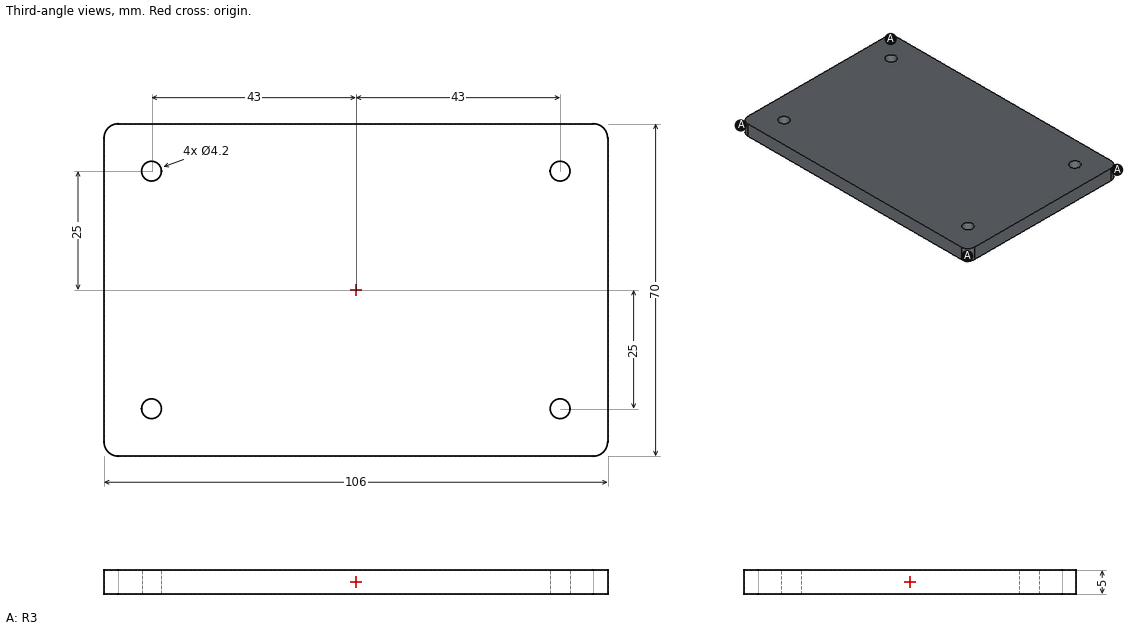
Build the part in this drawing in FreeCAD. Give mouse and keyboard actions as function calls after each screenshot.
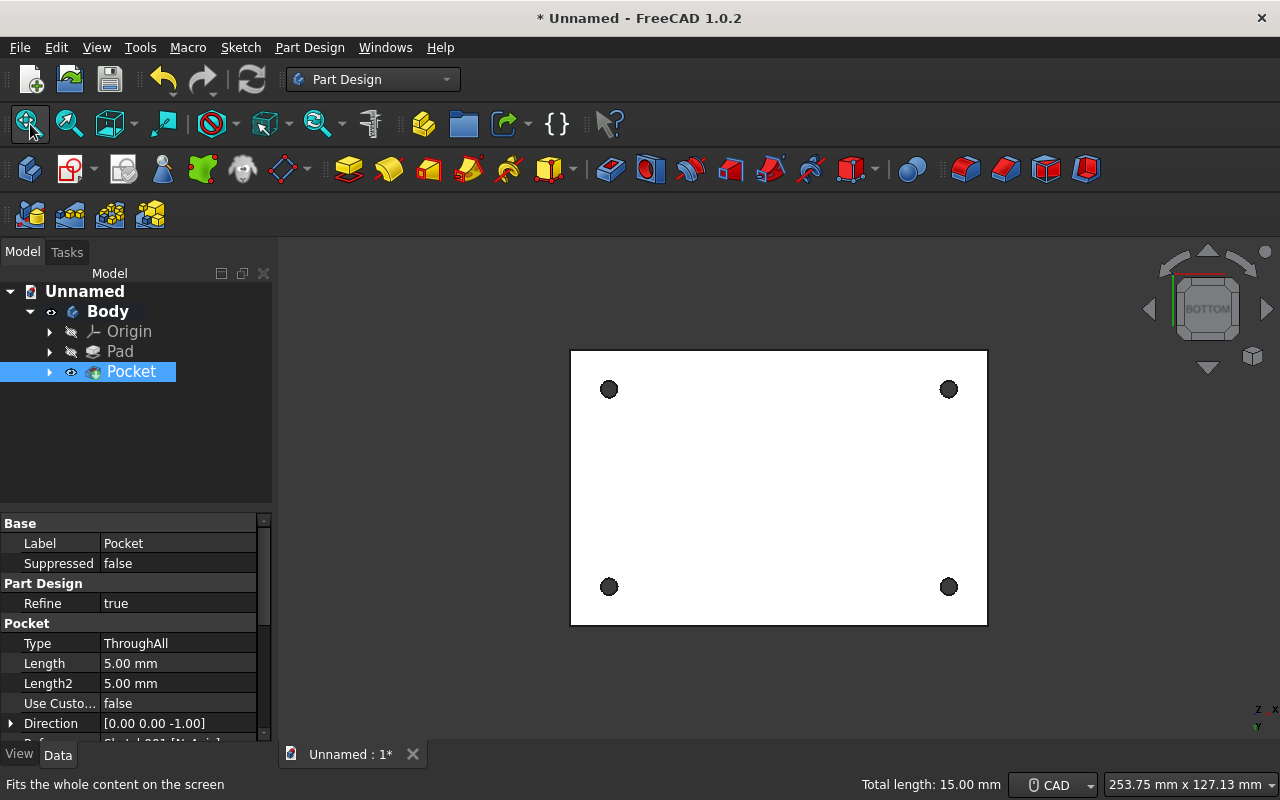
key(4)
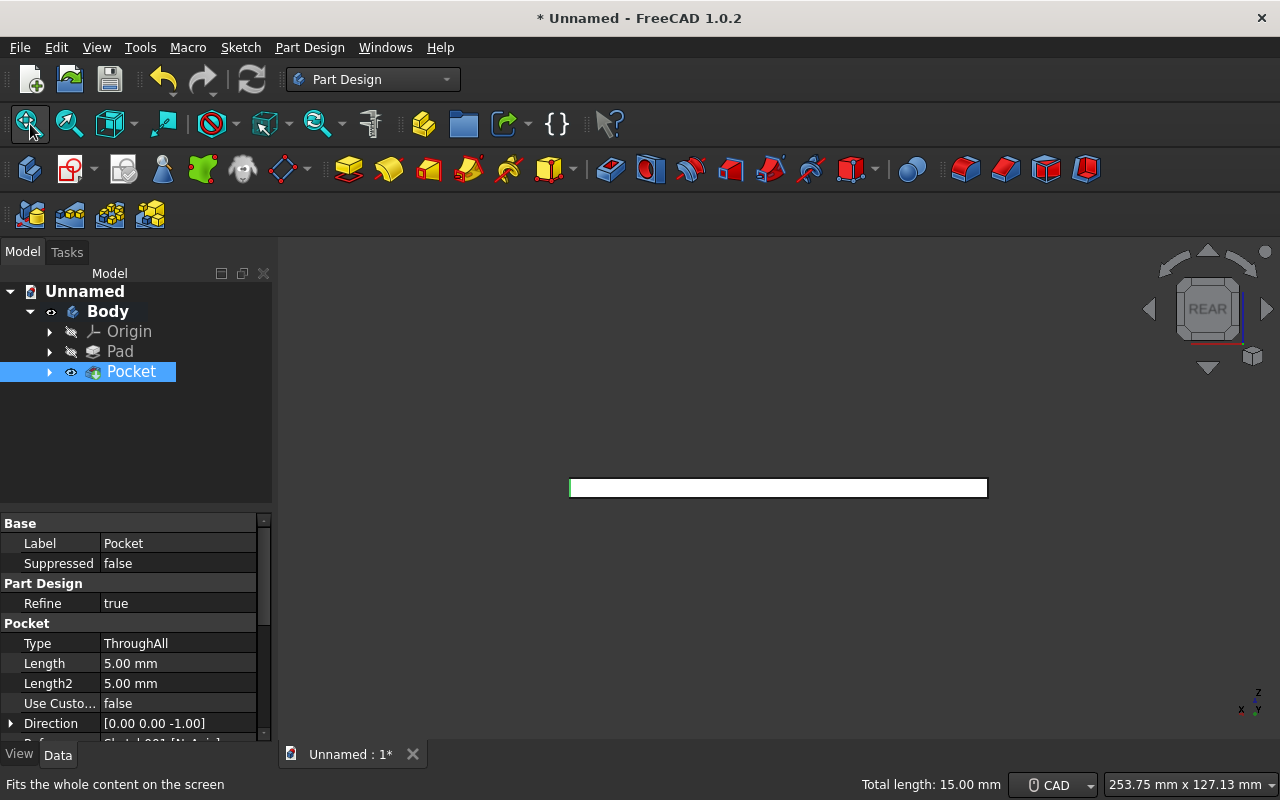
click(30, 124)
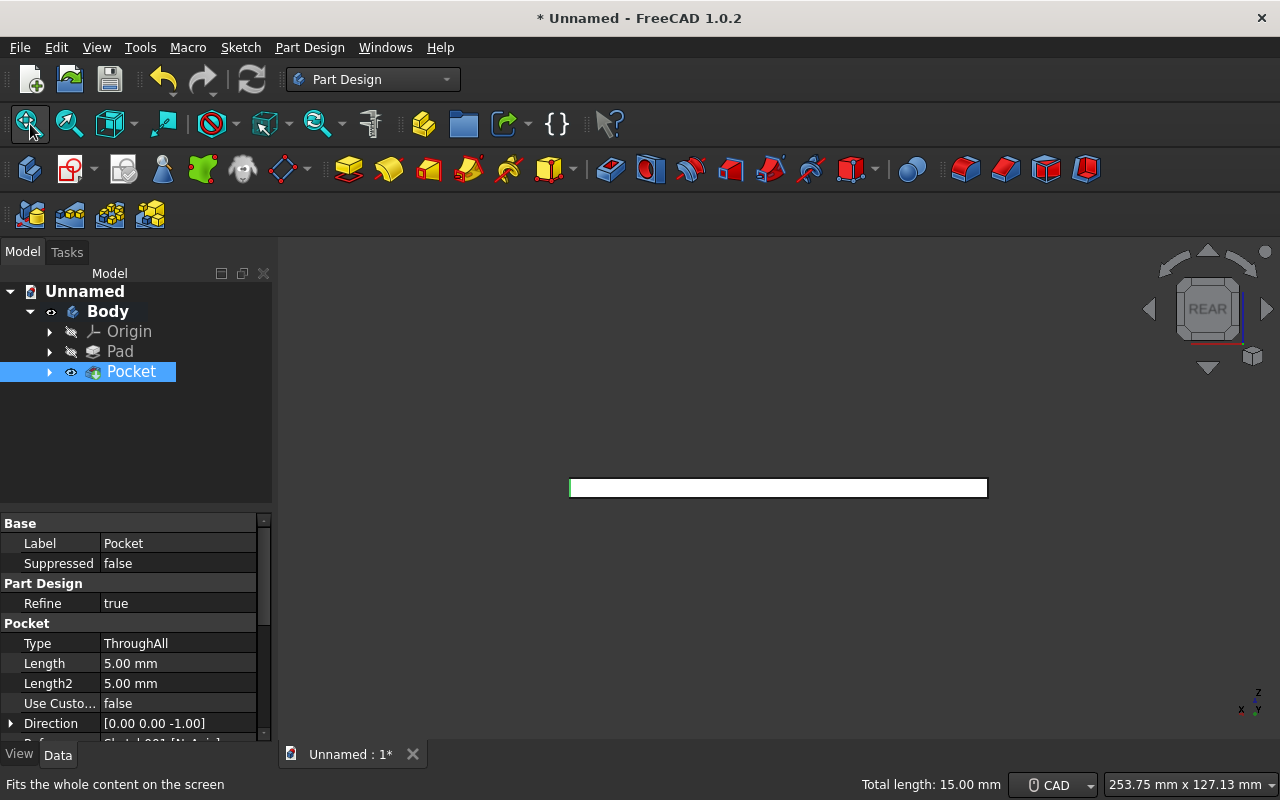
click(988, 487, ctrl)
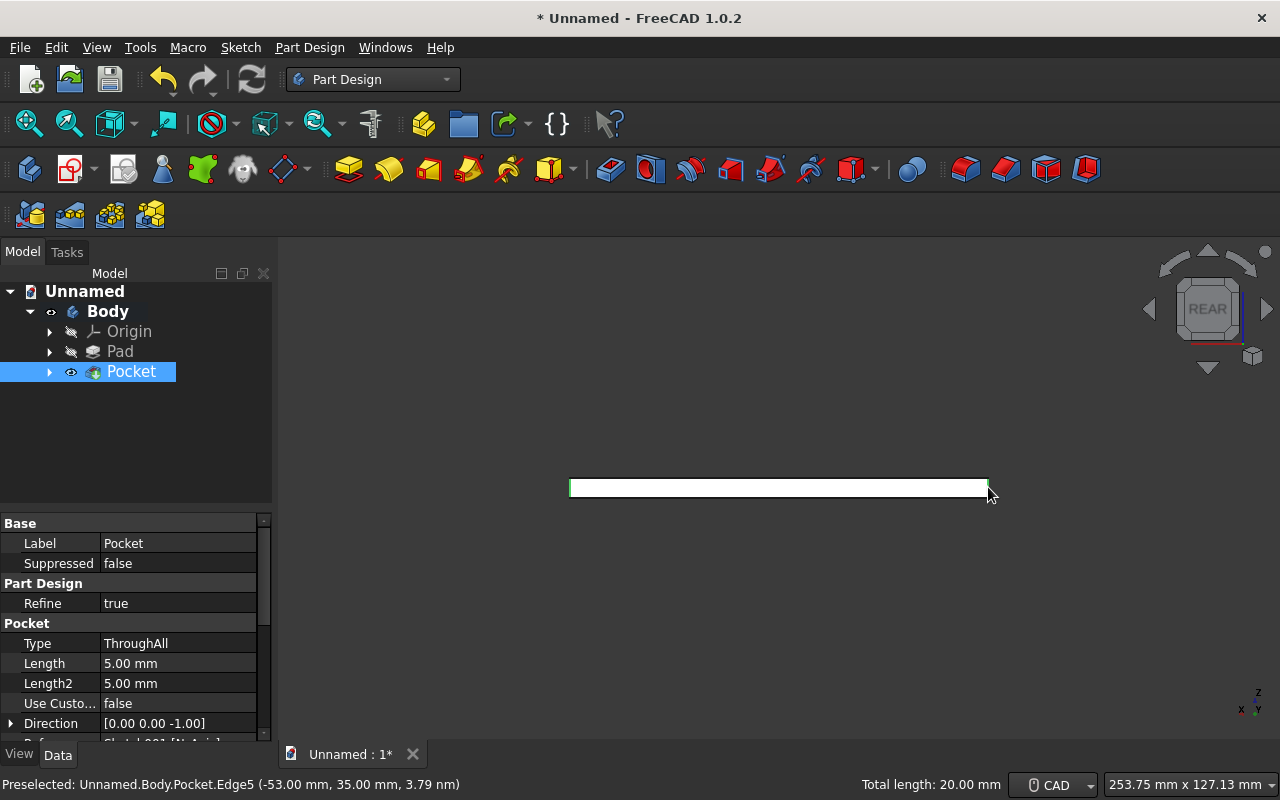
click(966, 170)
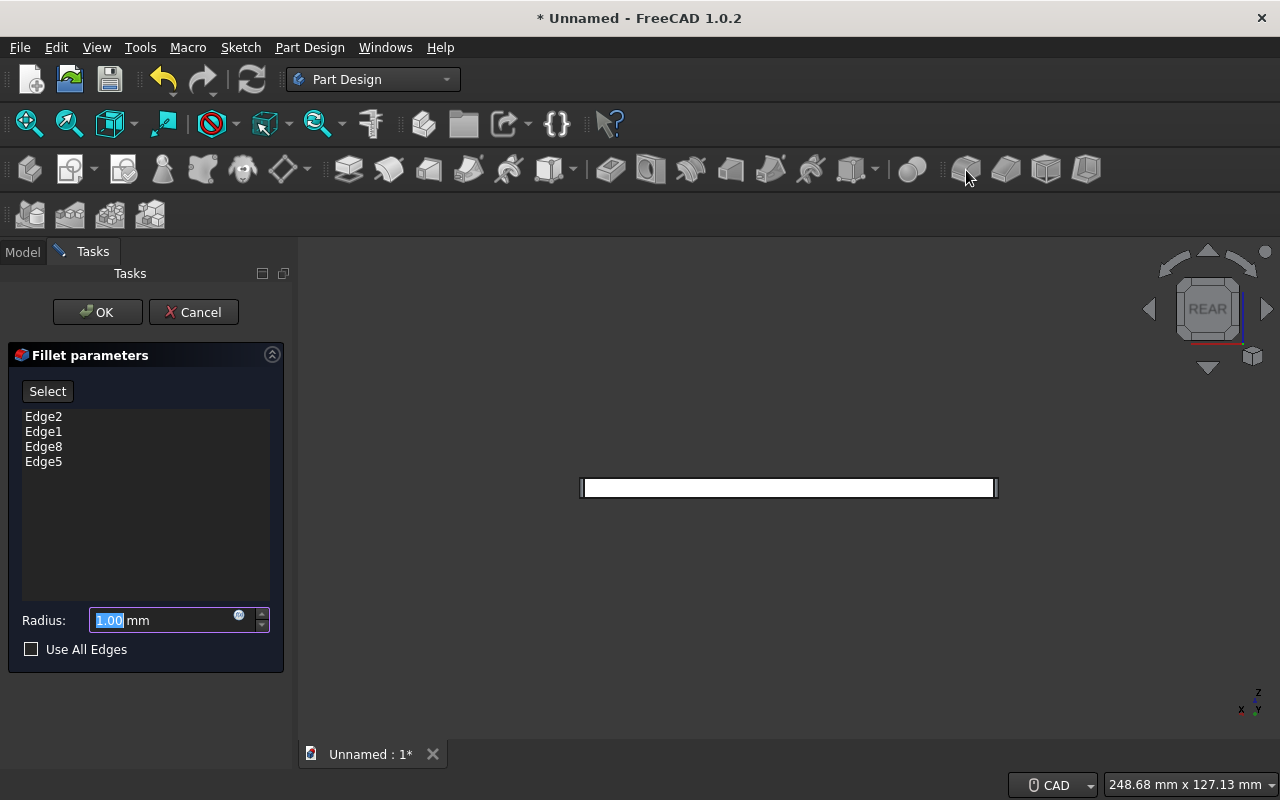
text(3)
key(Tab)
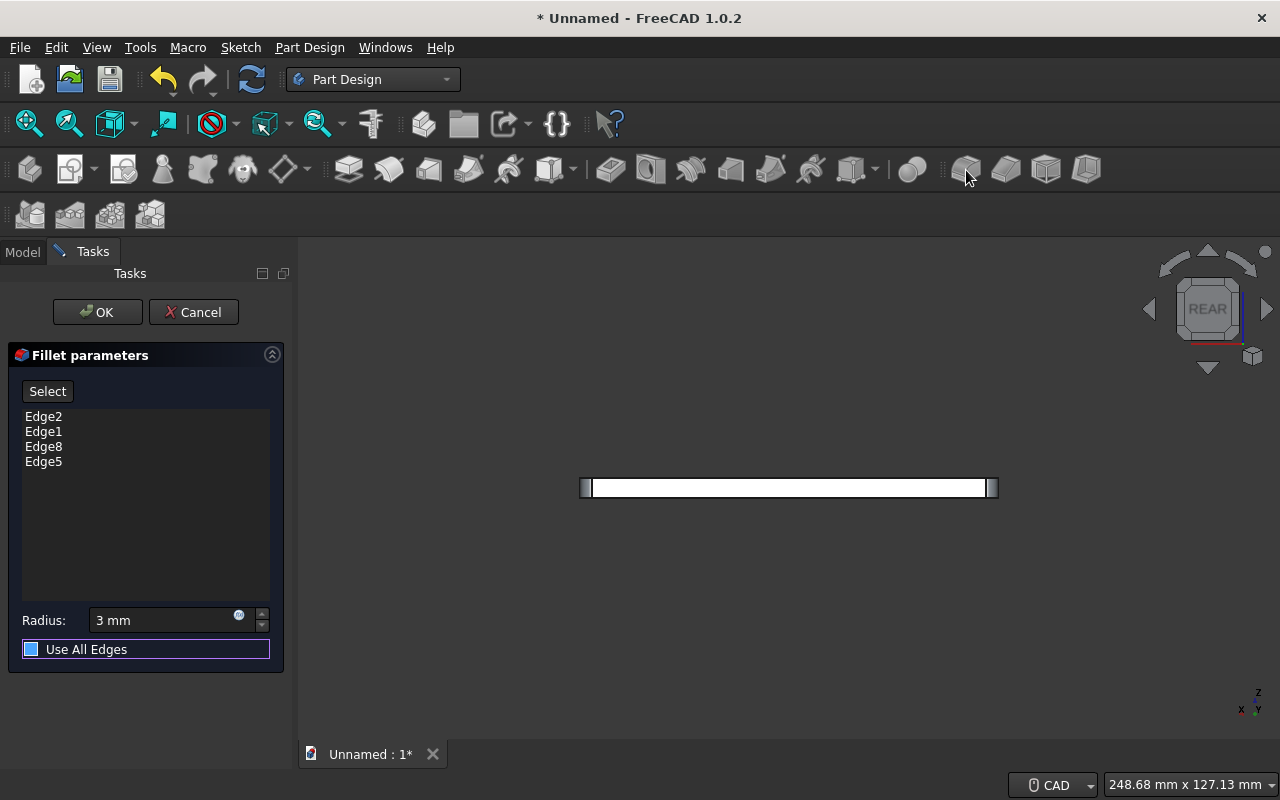
click(98, 312)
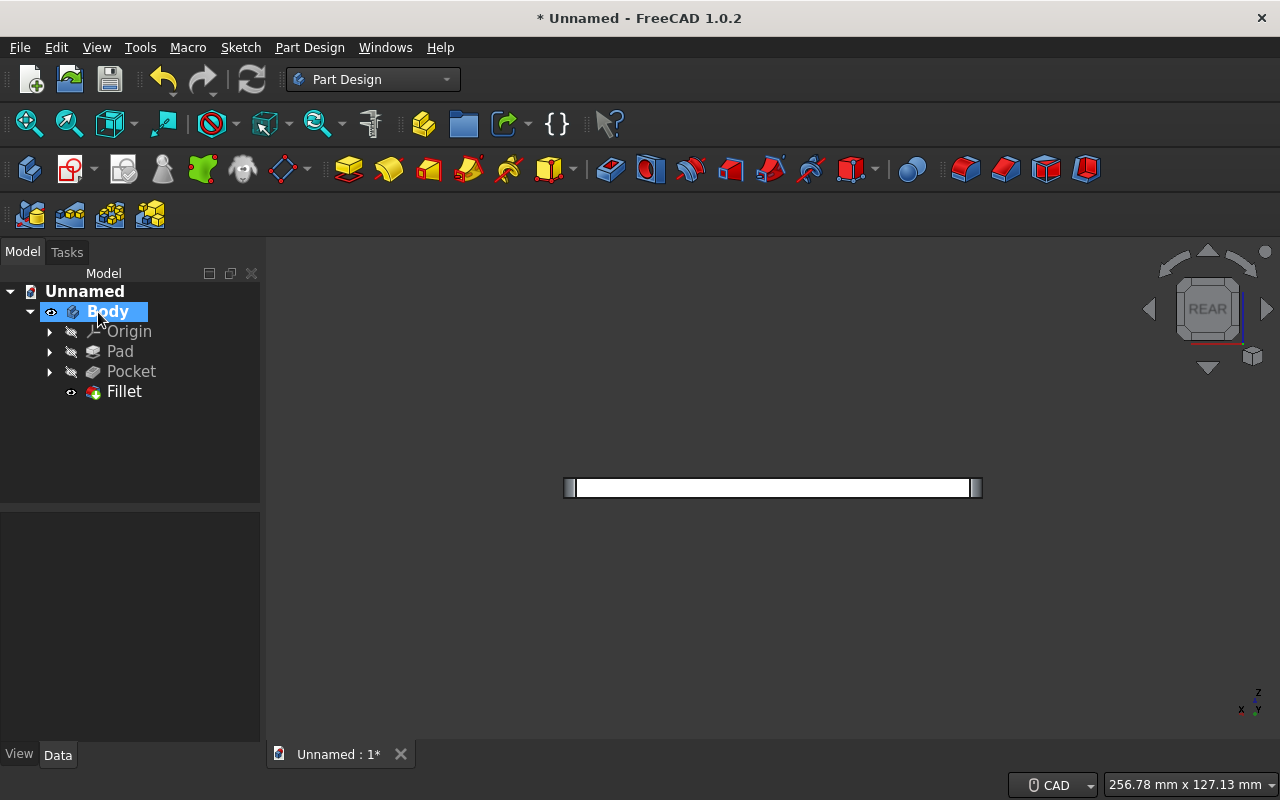
key(0)